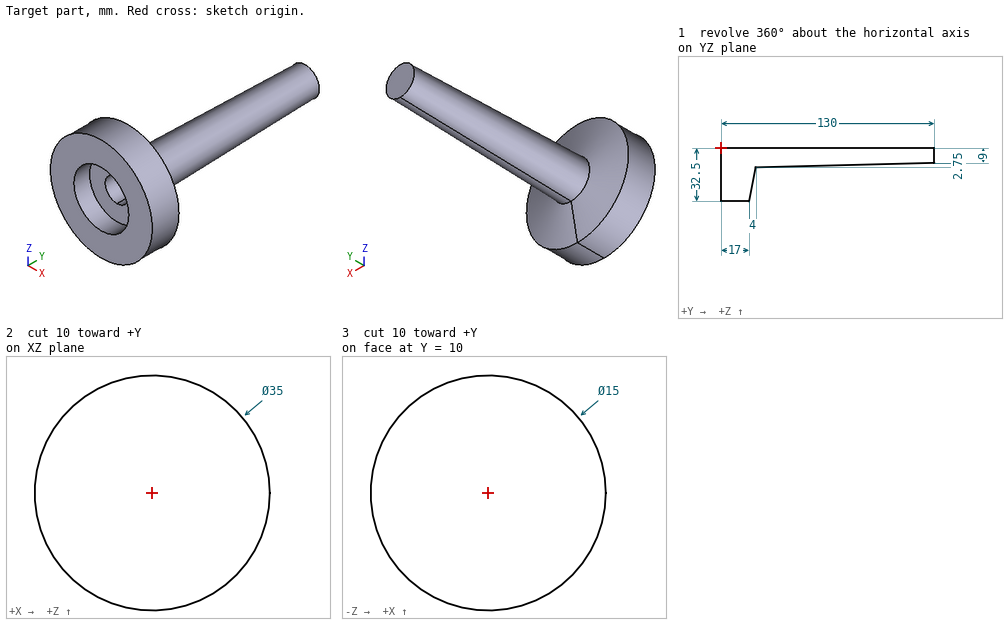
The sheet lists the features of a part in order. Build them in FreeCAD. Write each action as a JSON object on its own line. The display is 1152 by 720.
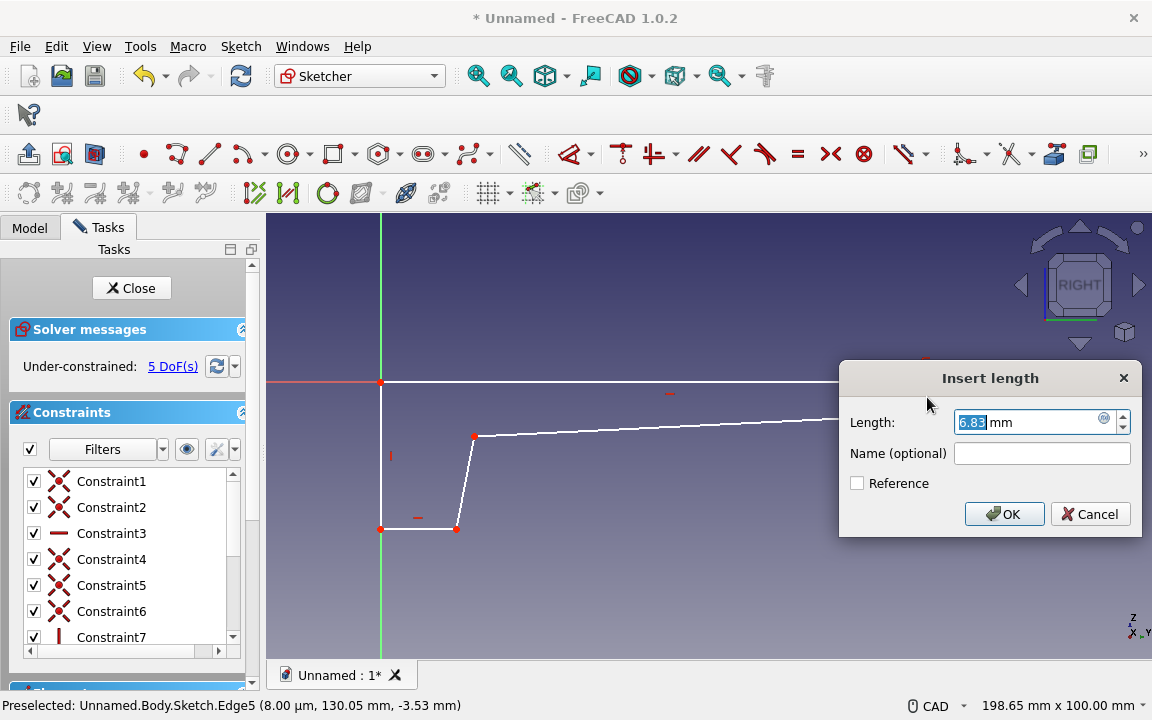
{"action": "type", "text": "9"}
{"action": "key", "text": "Return"}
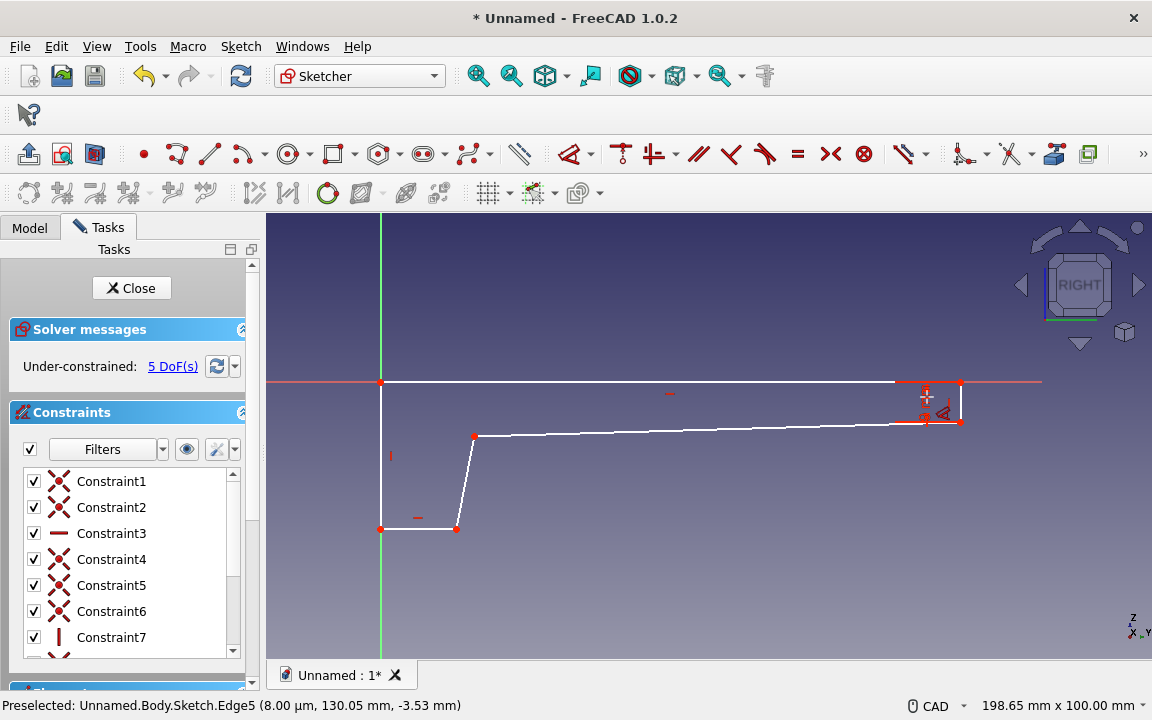
{"action": "left_click", "coordinate": [403, 529]}
{"action": "left_click", "coordinate": [418, 563]}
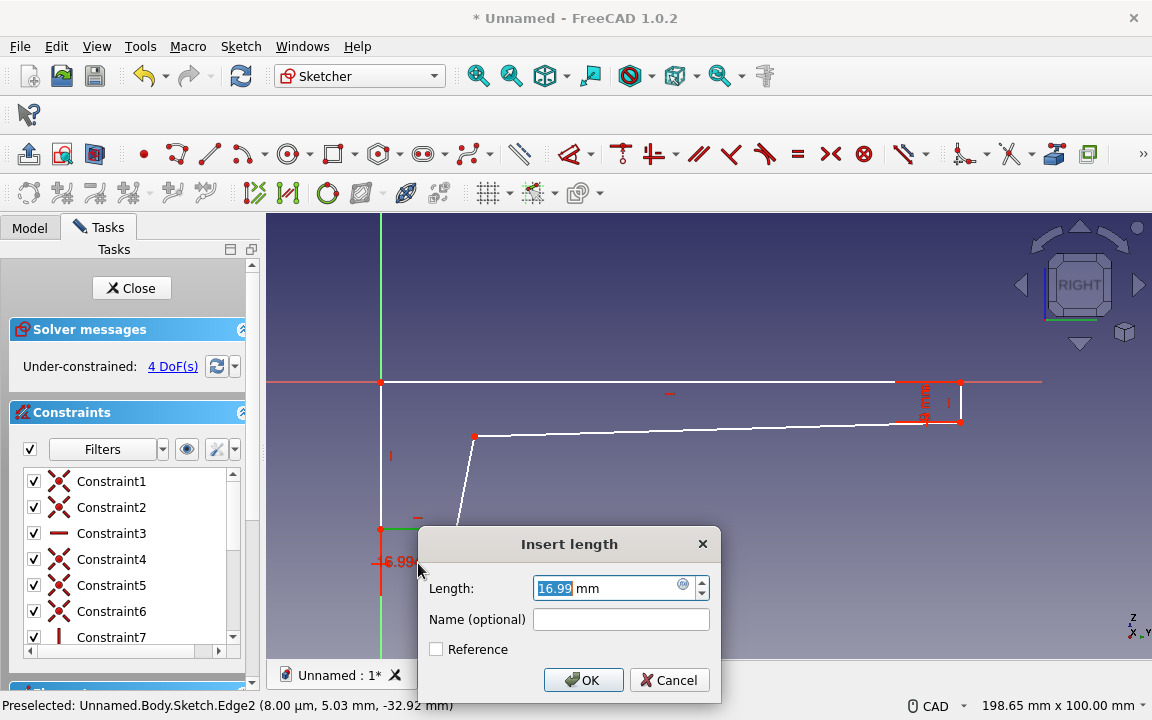
{"action": "type", "text": "17"}
{"action": "key", "text": "Return"}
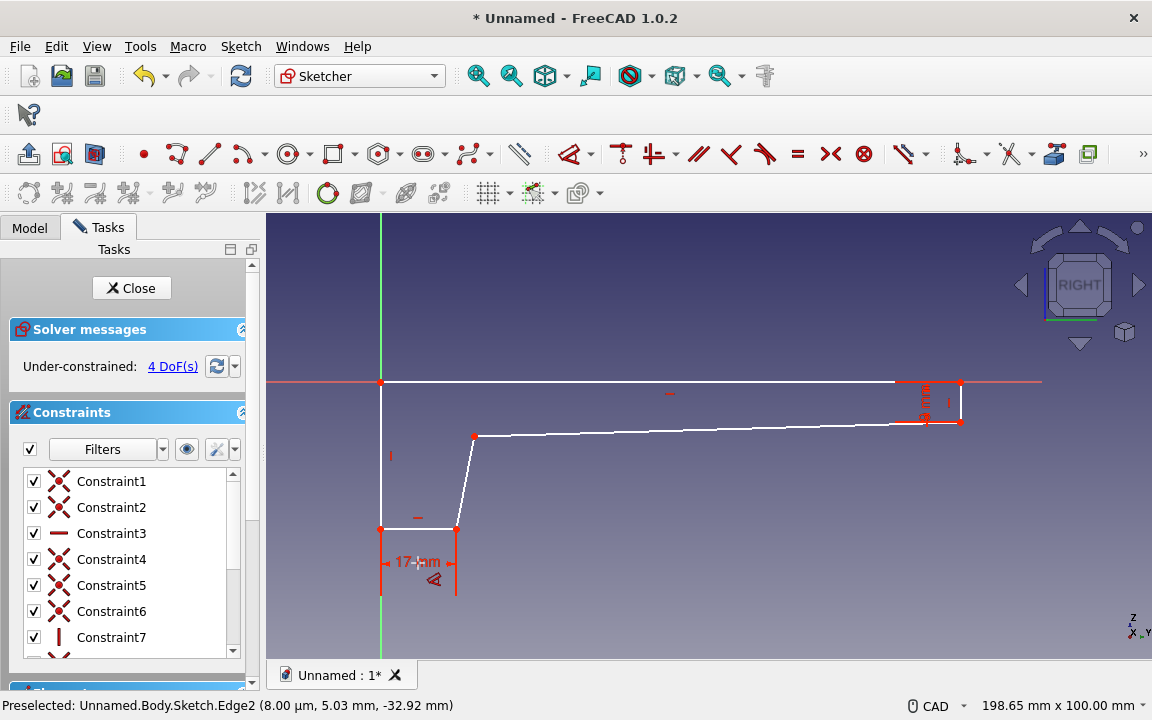
{"action": "scroll", "coordinate": [462, 501], "scroll_direction": "up", "scroll_amount": 4}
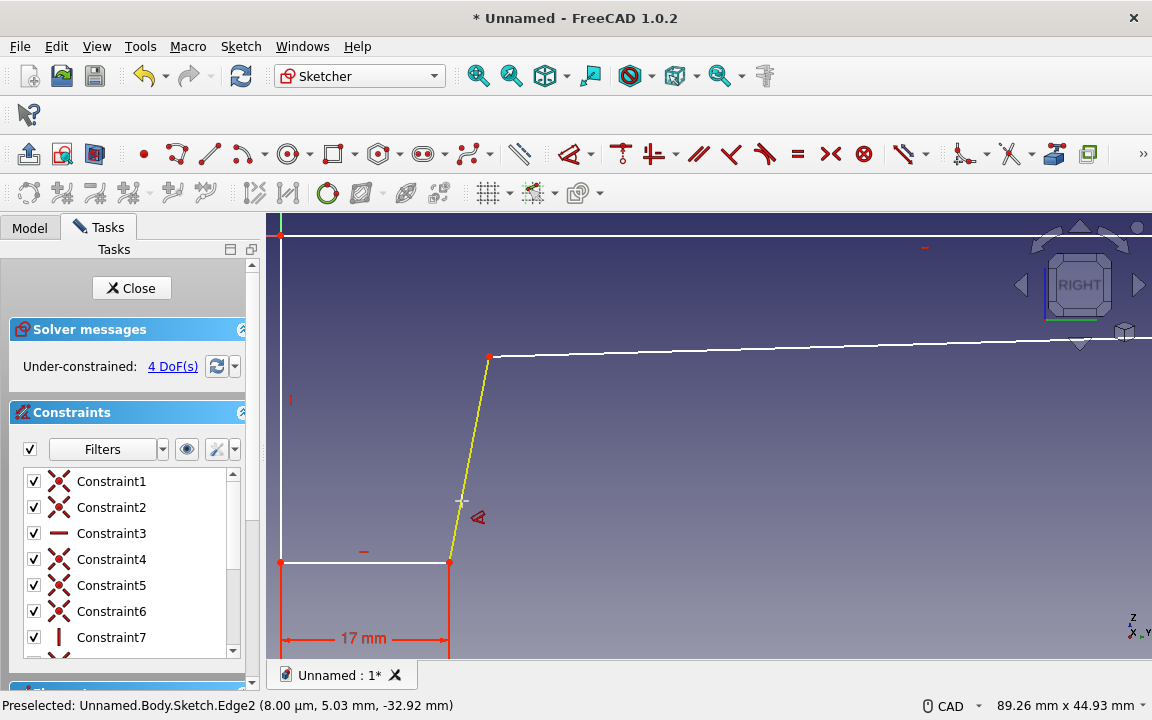
{"action": "left_click", "coordinate": [461, 501]}
{"action": "left_click", "coordinate": [469, 597]}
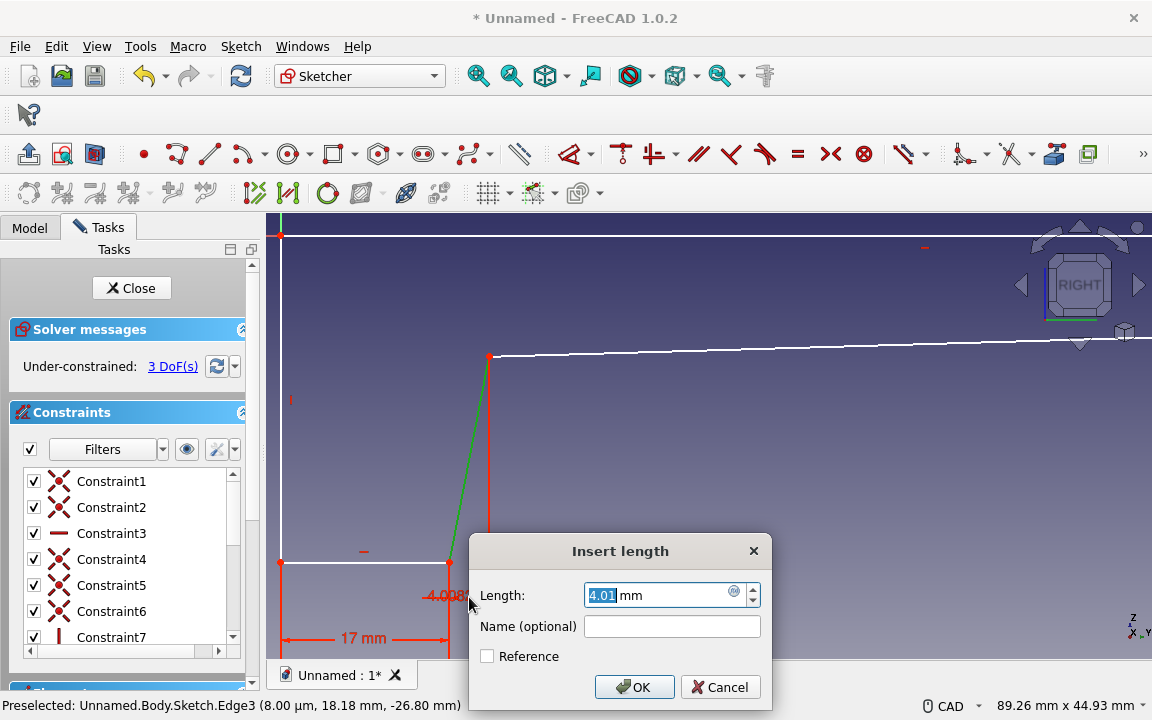
{"action": "type", "text": "4"}
{"action": "key", "text": "Return"}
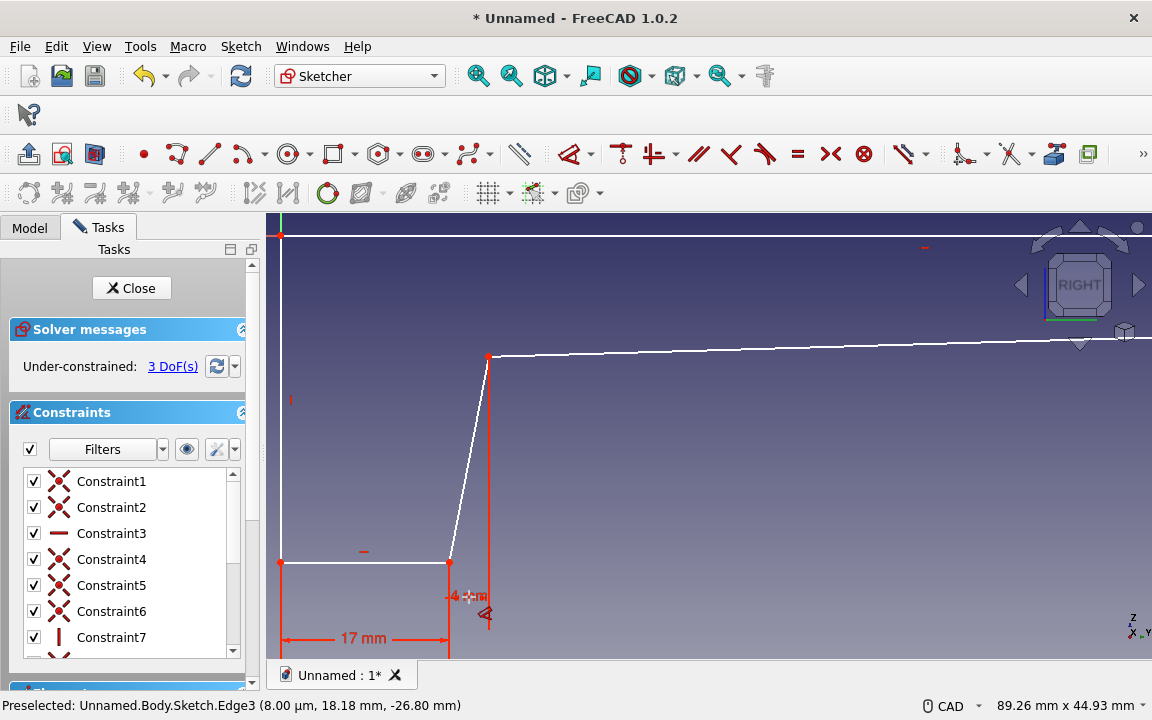
{"action": "scroll", "coordinate": [475, 459], "scroll_direction": "down", "scroll_amount": 5}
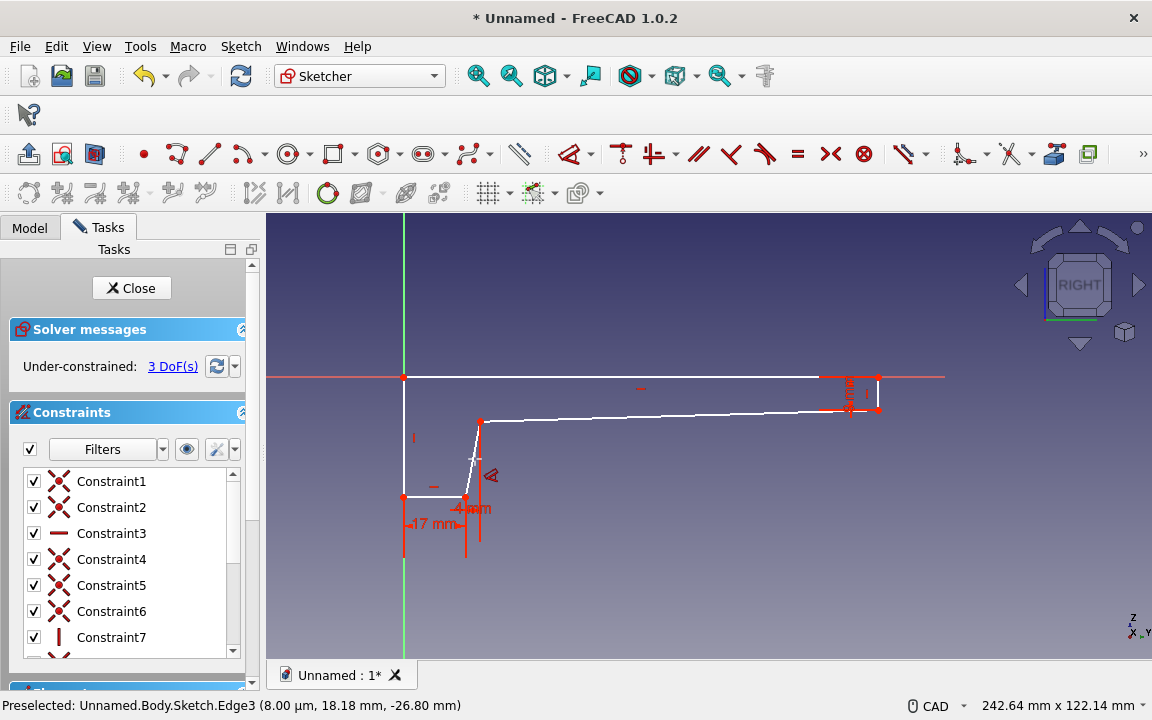
{"action": "left_click", "coordinate": [736, 377]}
{"action": "left_click", "coordinate": [641, 343]}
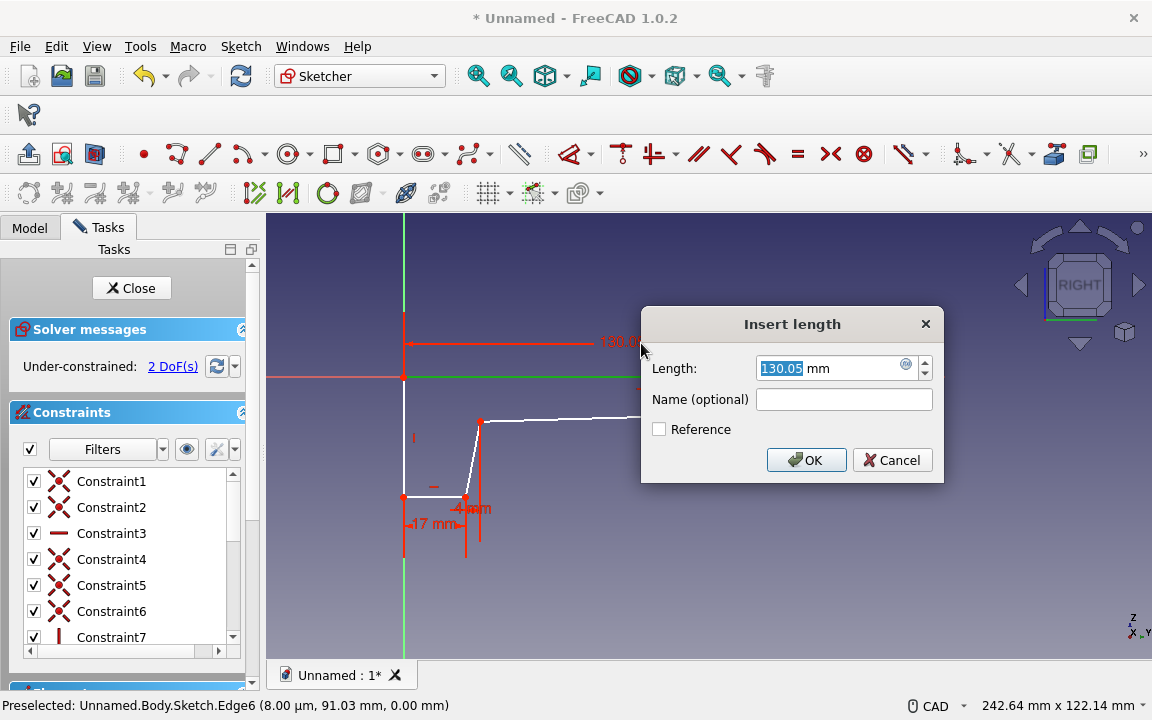
{"action": "type", "text": "130"}
{"action": "key", "text": "Return"}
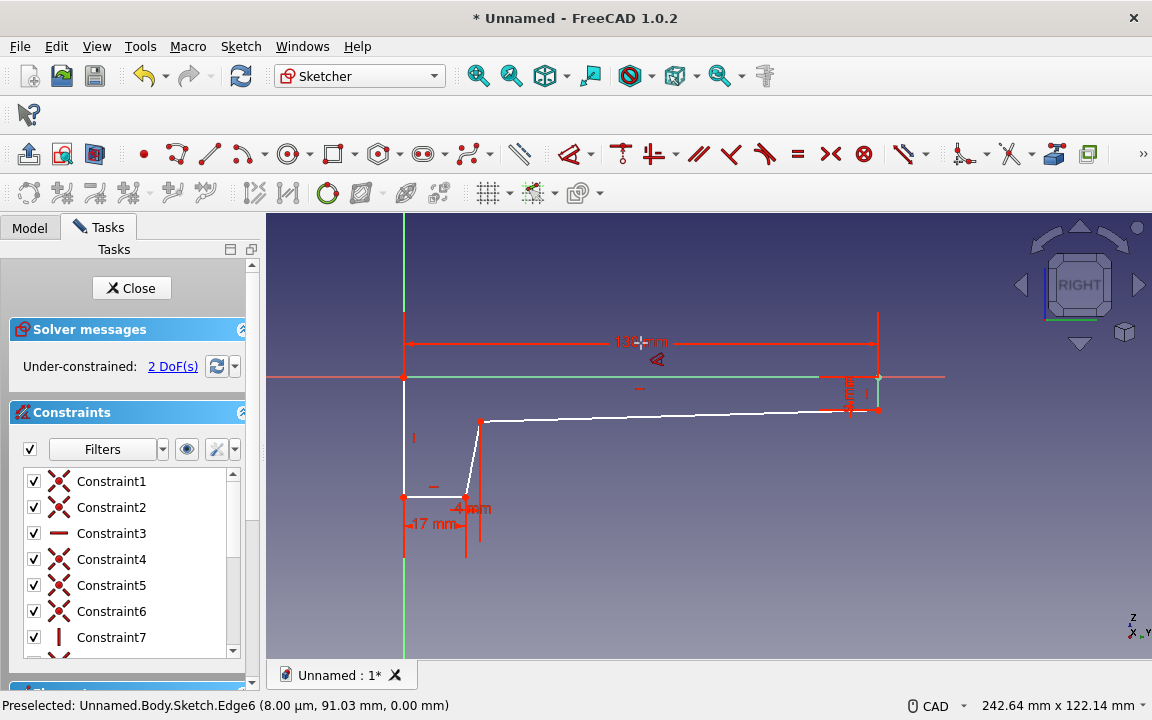
{"action": "left_click", "coordinate": [404, 413]}
{"action": "left_click", "coordinate": [370, 437]}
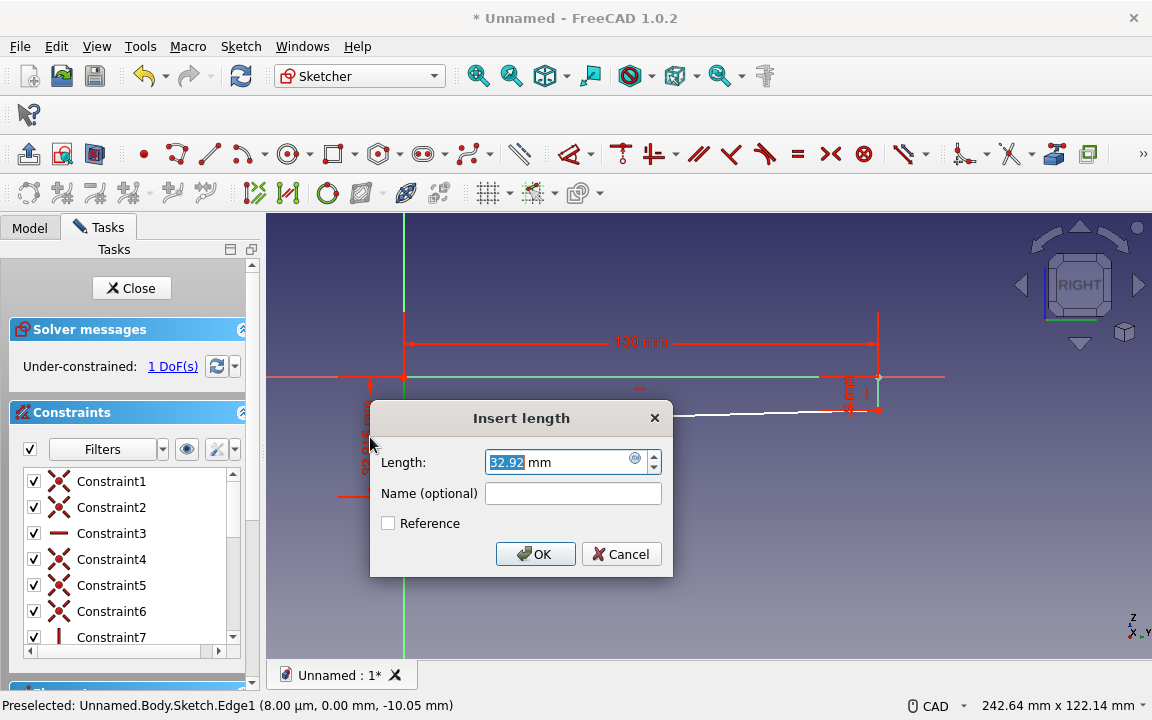
{"action": "type", "text": "32.5"}
{"action": "key", "text": "Return"}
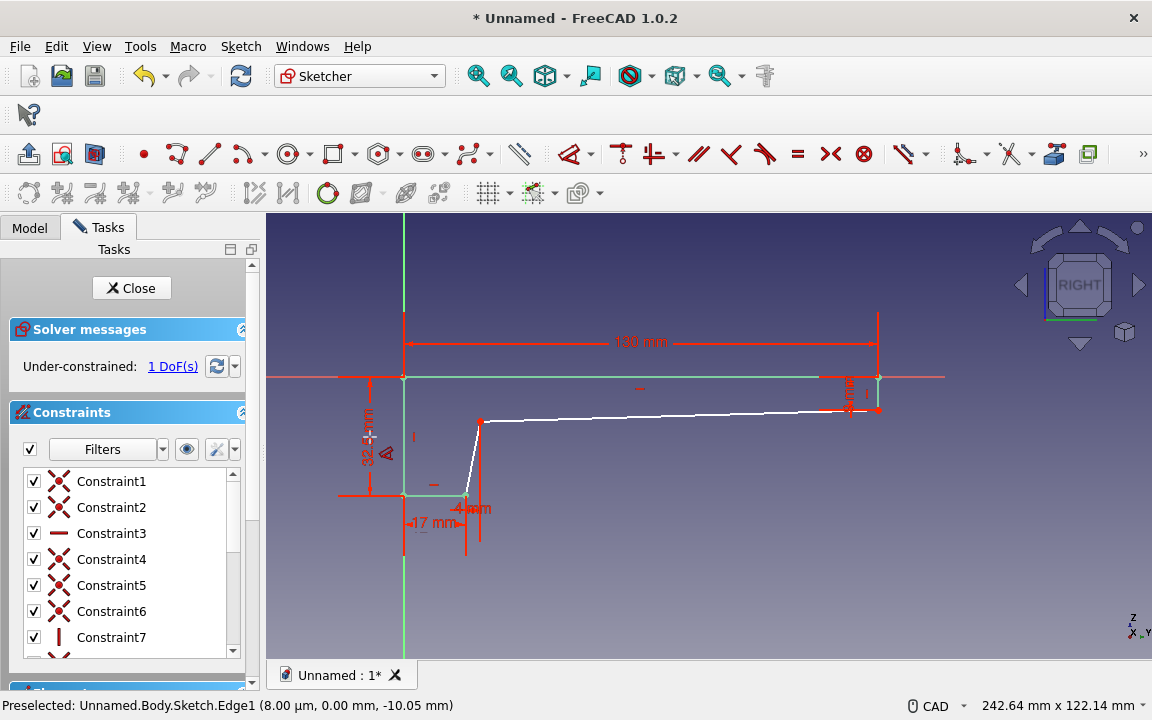
{"action": "scroll", "coordinate": [600, 418], "scroll_direction": "up", "scroll_amount": 7}